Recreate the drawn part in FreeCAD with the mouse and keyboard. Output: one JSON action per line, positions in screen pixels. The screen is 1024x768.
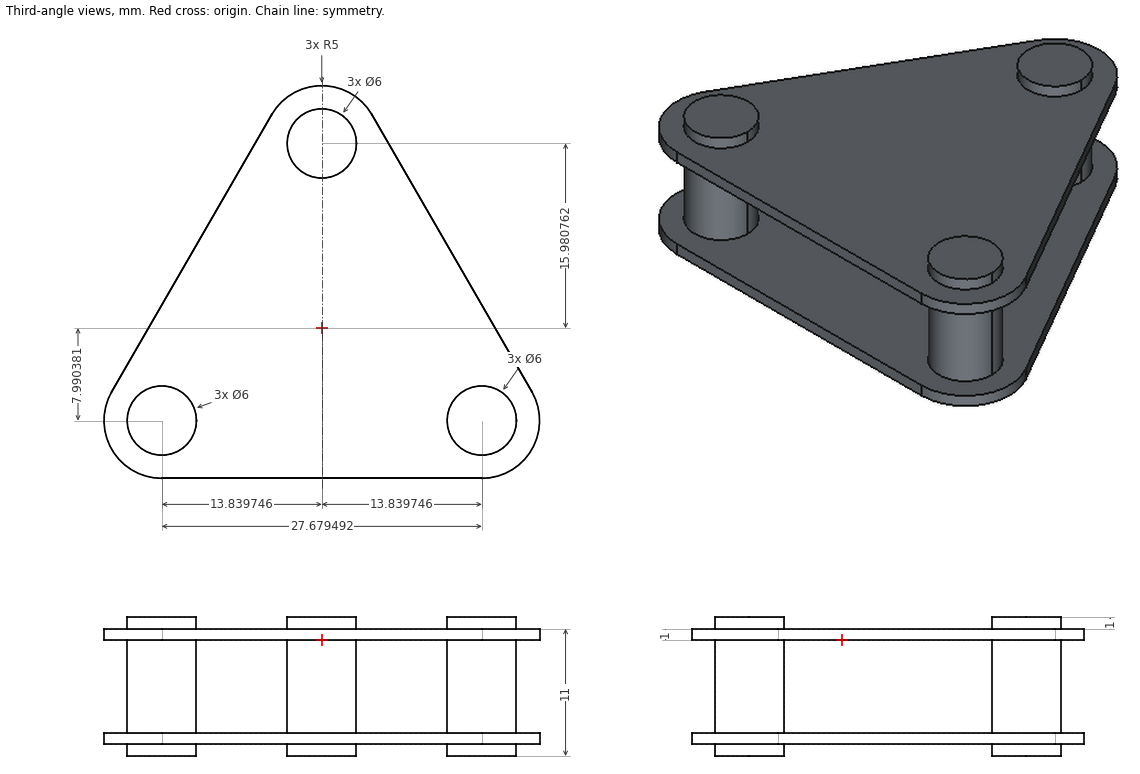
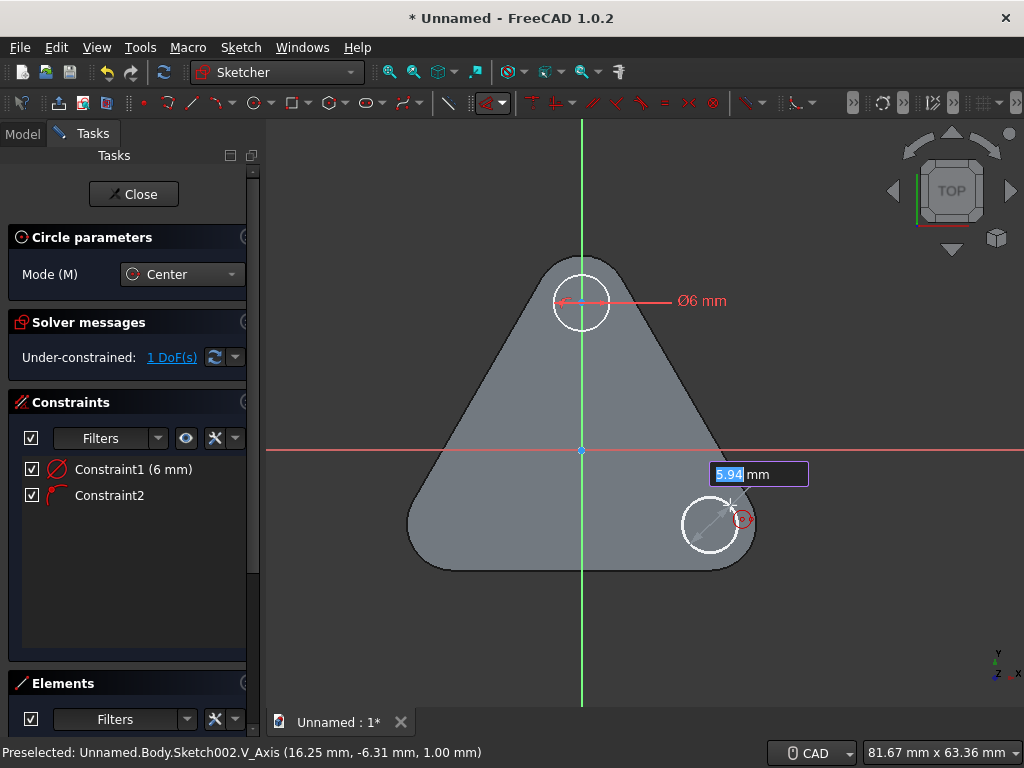
{"action": "type", "text": "6"}
{"action": "key", "text": "Return"}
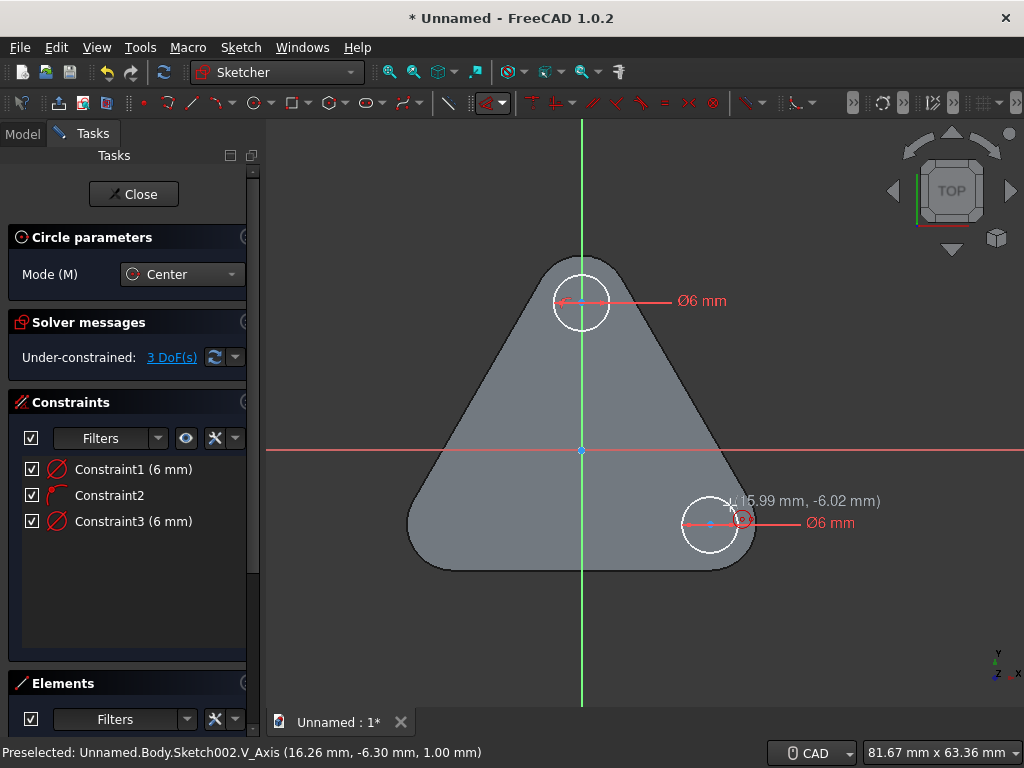
{"action": "left_click", "coordinate": [453, 524]}
{"action": "mouse_move", "coordinate": [473, 505]}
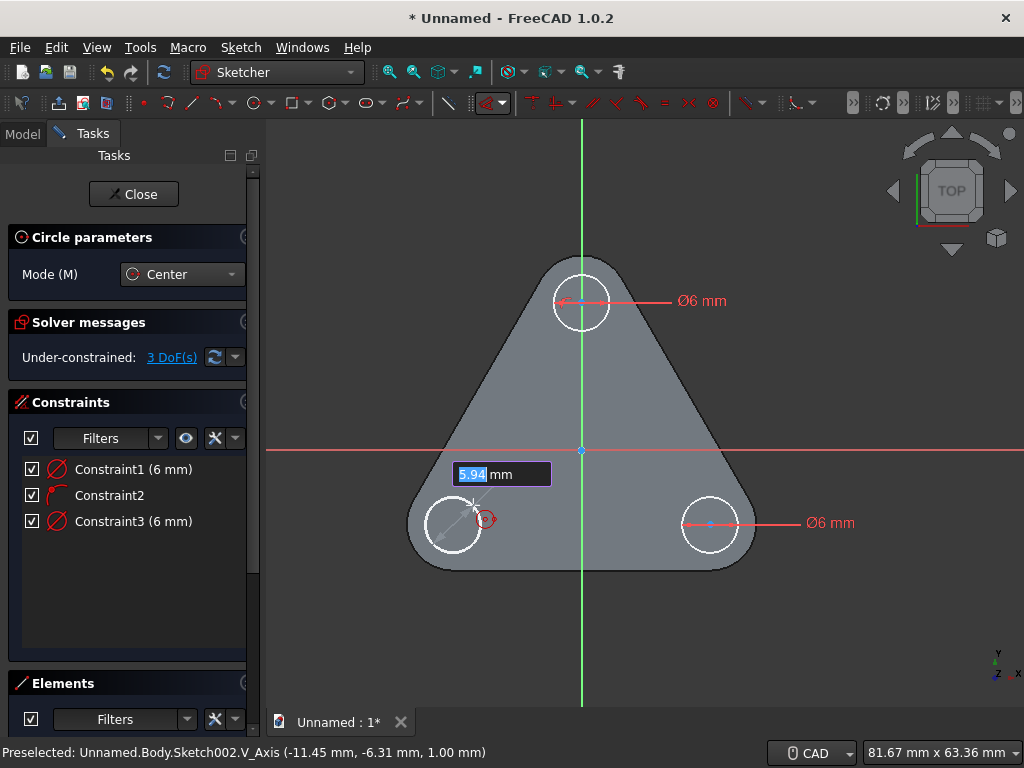
{"action": "type", "text": "6"}
{"action": "key", "text": "Return"}
{"action": "key", "text": "Escape"}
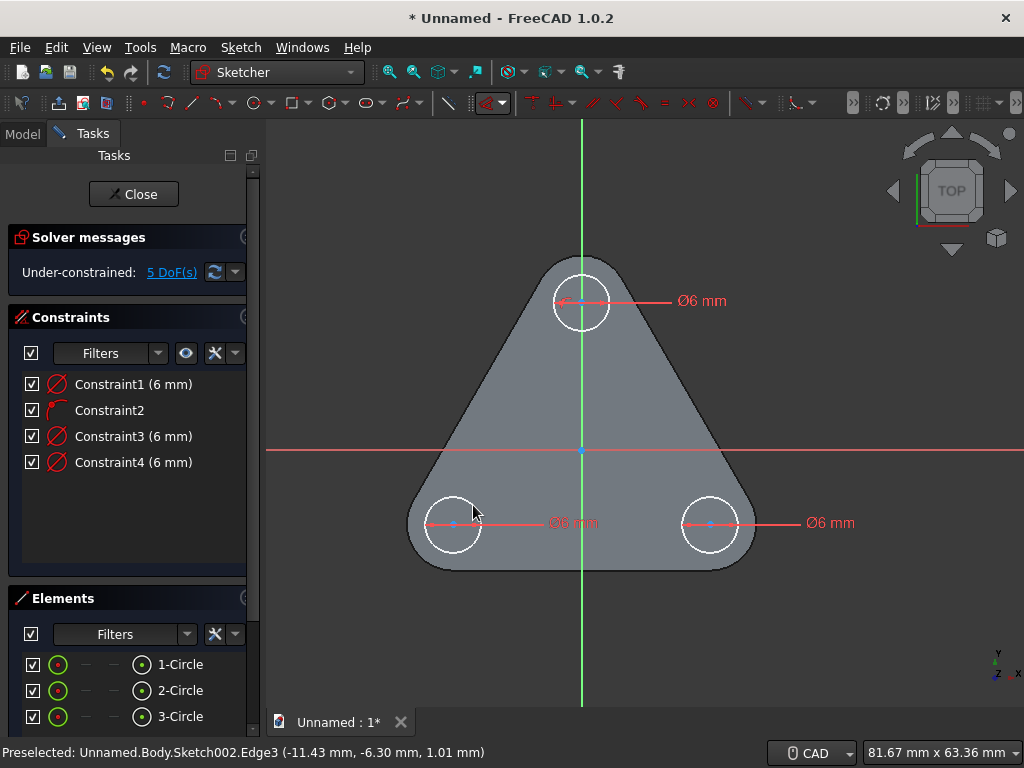
{"action": "left_click", "coordinate": [710, 525]}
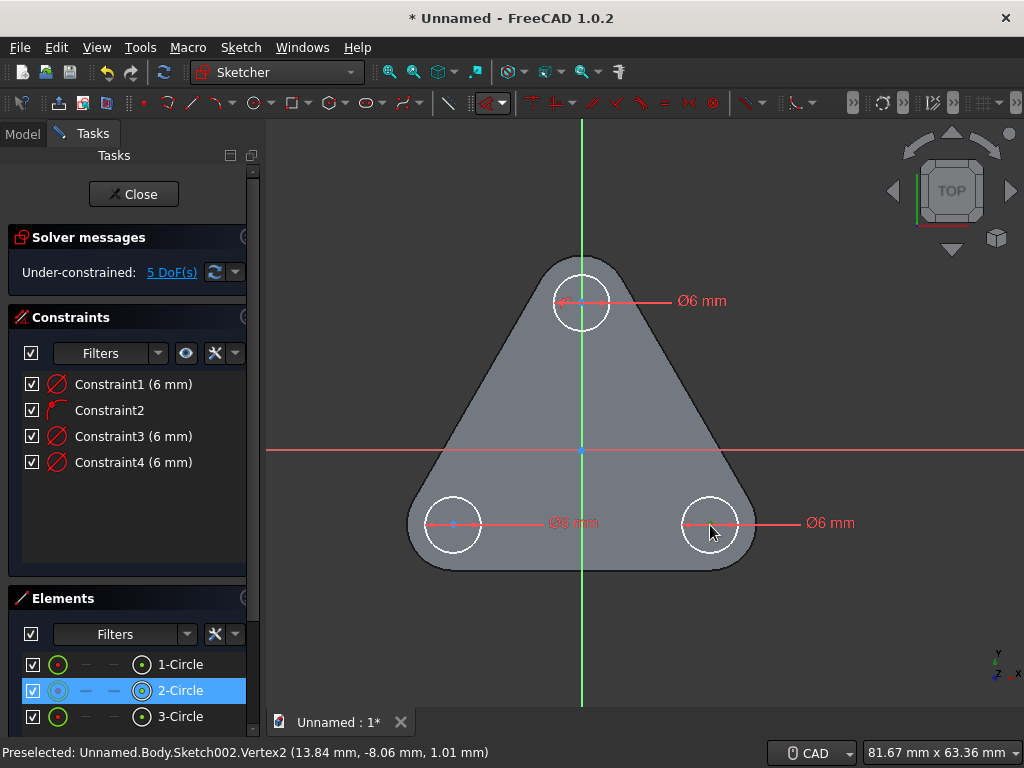
{"action": "left_click", "coordinate": [453, 525]}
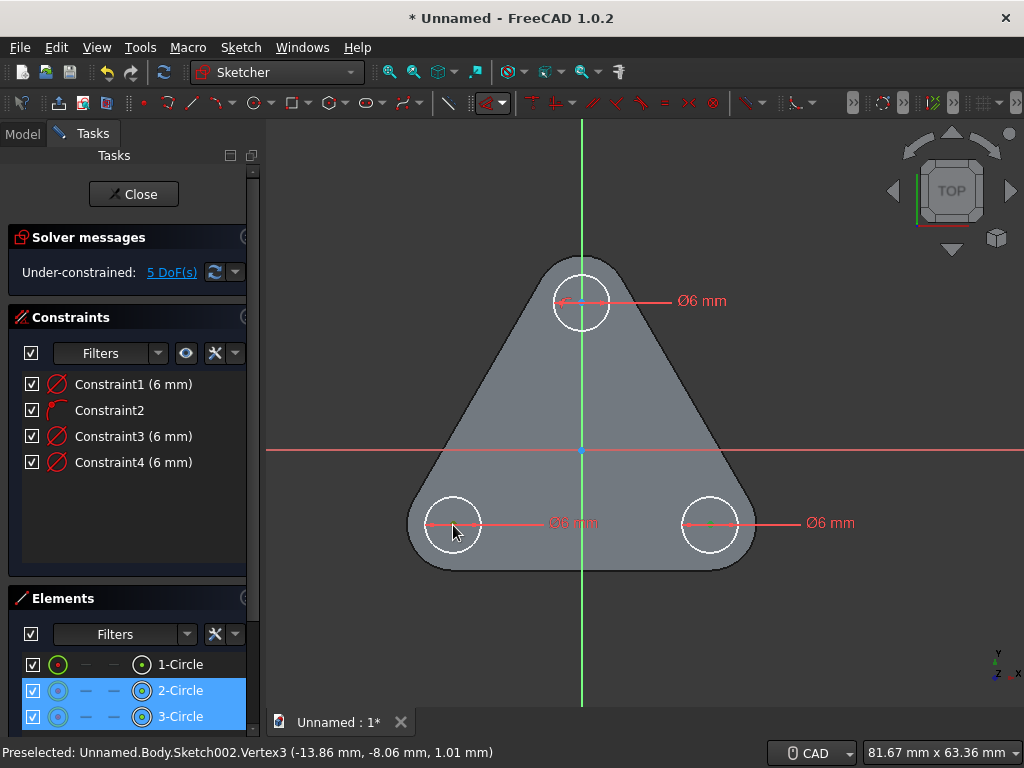
{"action": "left_click", "coordinate": [582, 641]}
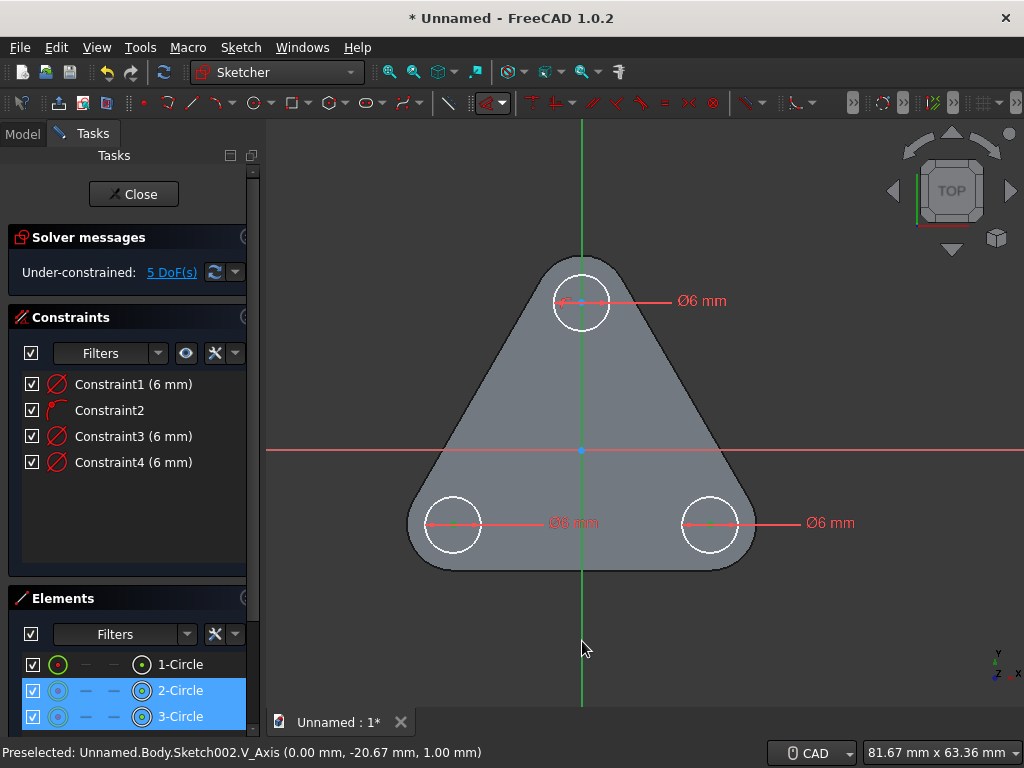
{"action": "left_click", "coordinate": [690, 104]}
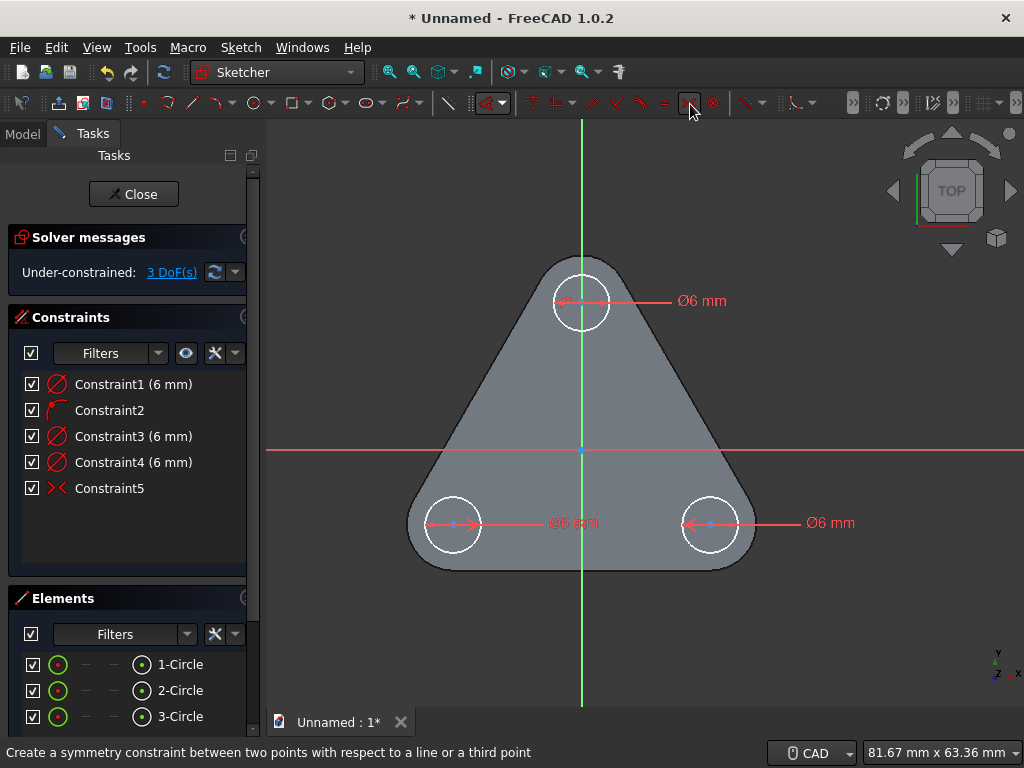
{"action": "left_click", "coordinate": [710, 525]}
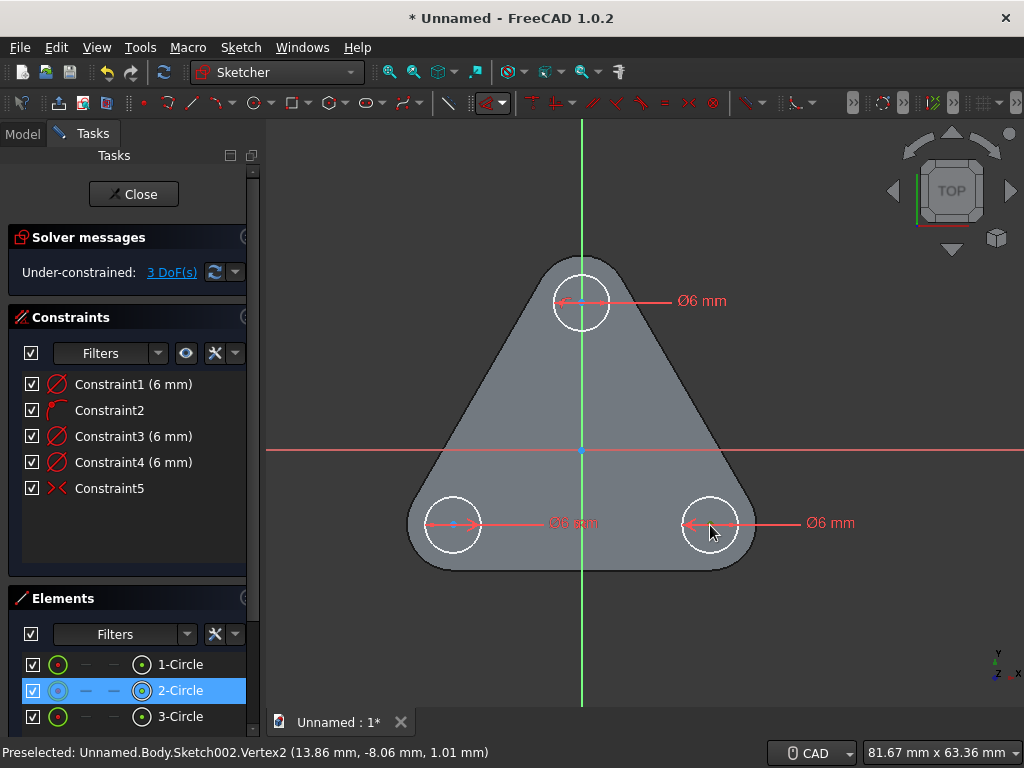
{"action": "key", "text": "i"}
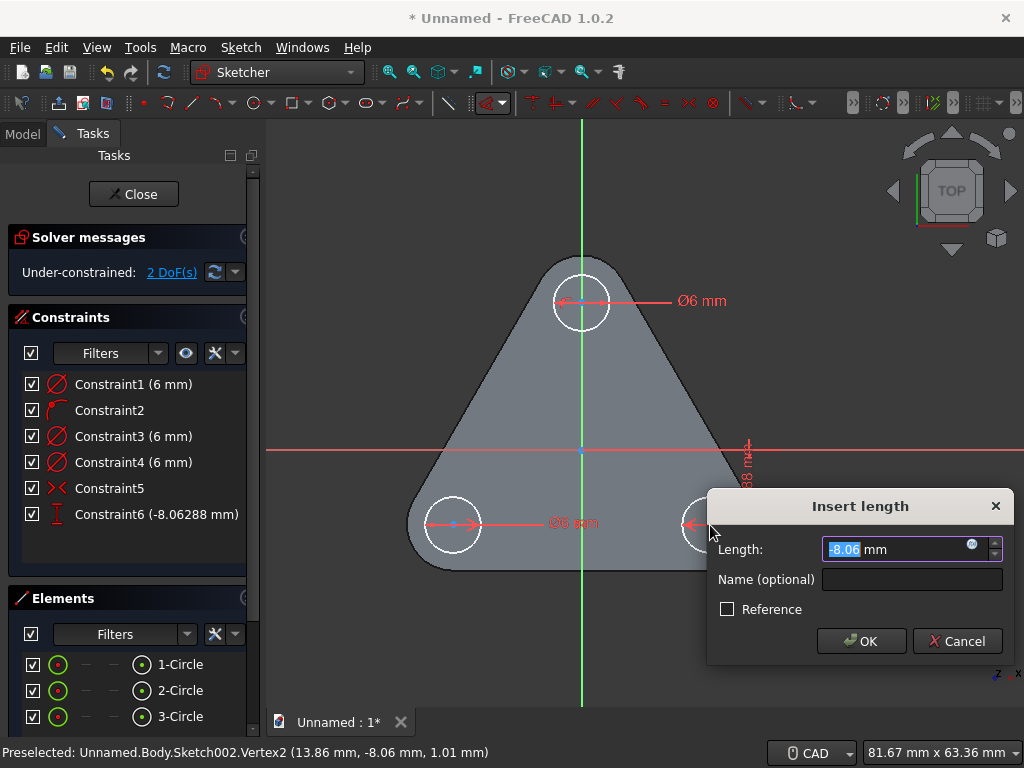
{"action": "type", "text": "-7.990381"}
{"action": "key", "text": "Return"}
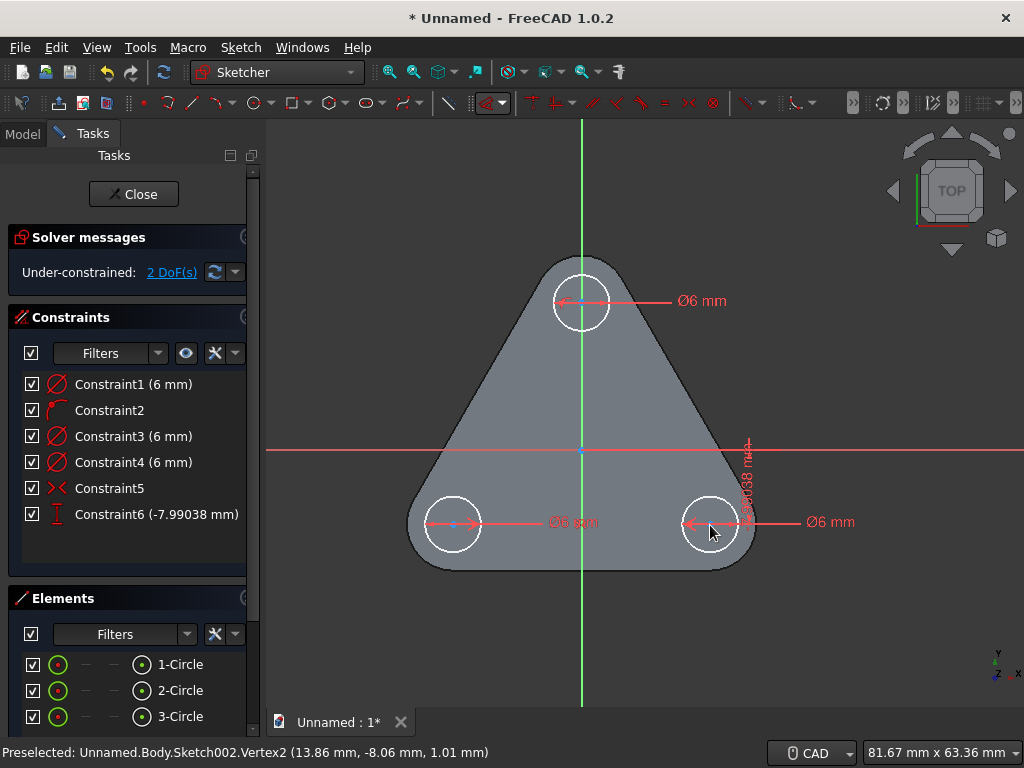
{"action": "left_click", "coordinate": [582, 303]}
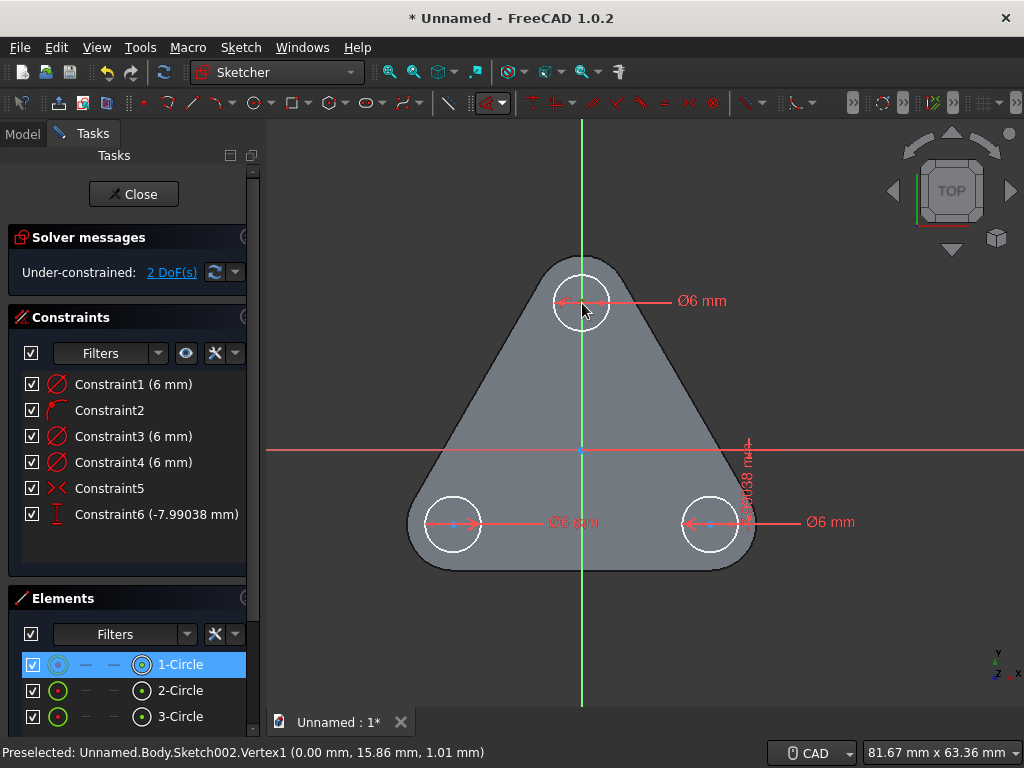
{"action": "left_click", "coordinate": [504, 104]}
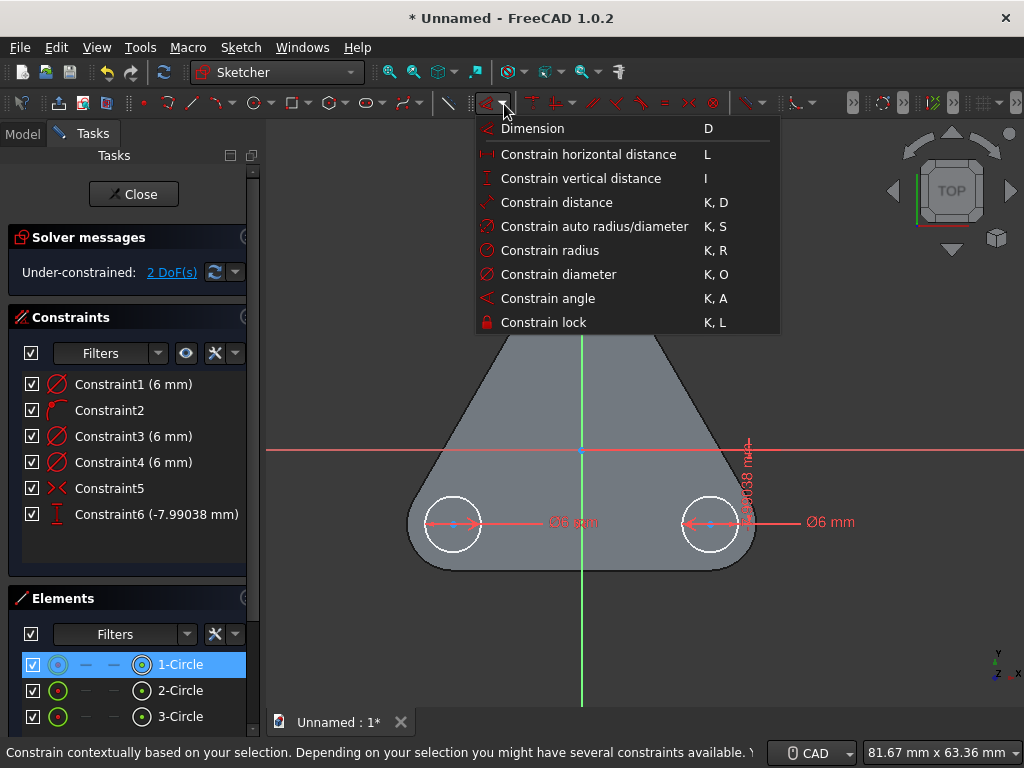
{"action": "left_click", "coordinate": [628, 178]}